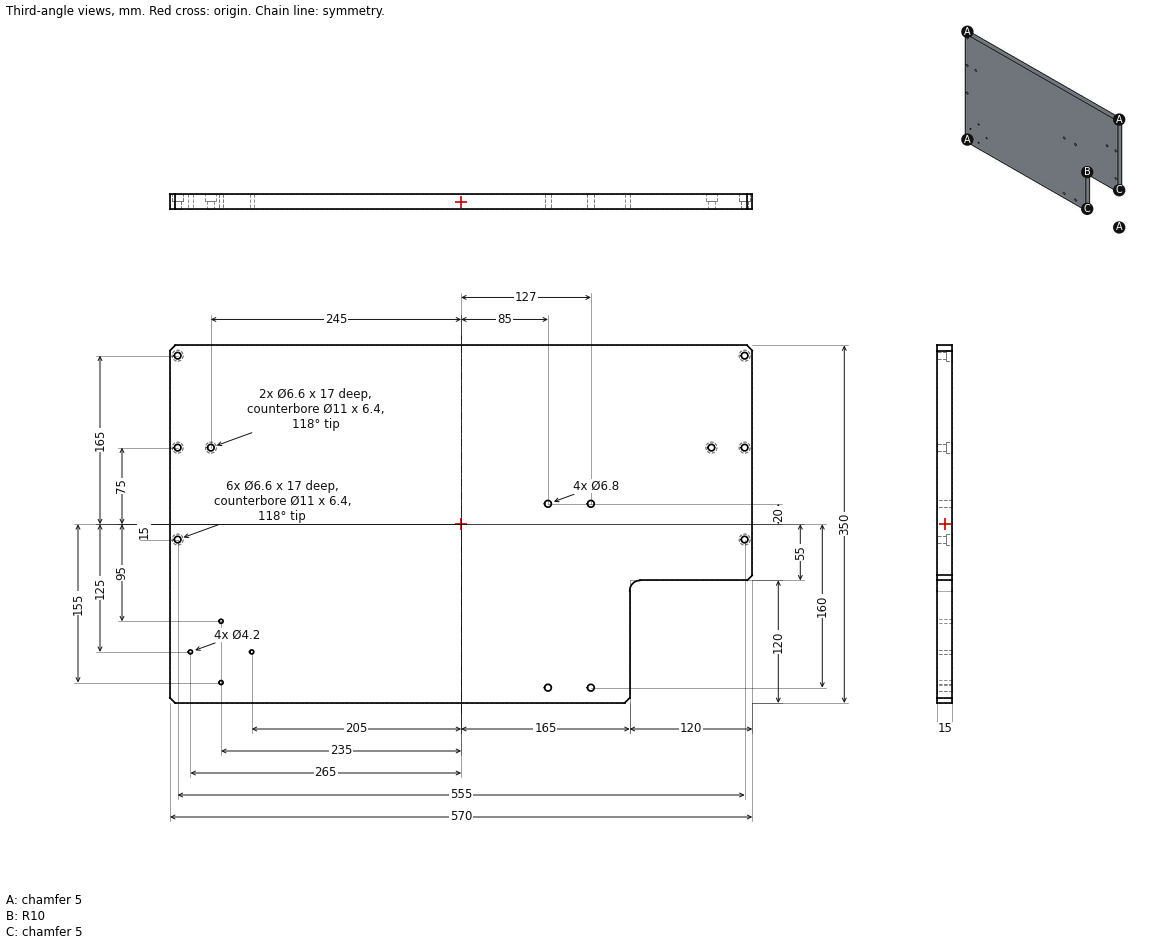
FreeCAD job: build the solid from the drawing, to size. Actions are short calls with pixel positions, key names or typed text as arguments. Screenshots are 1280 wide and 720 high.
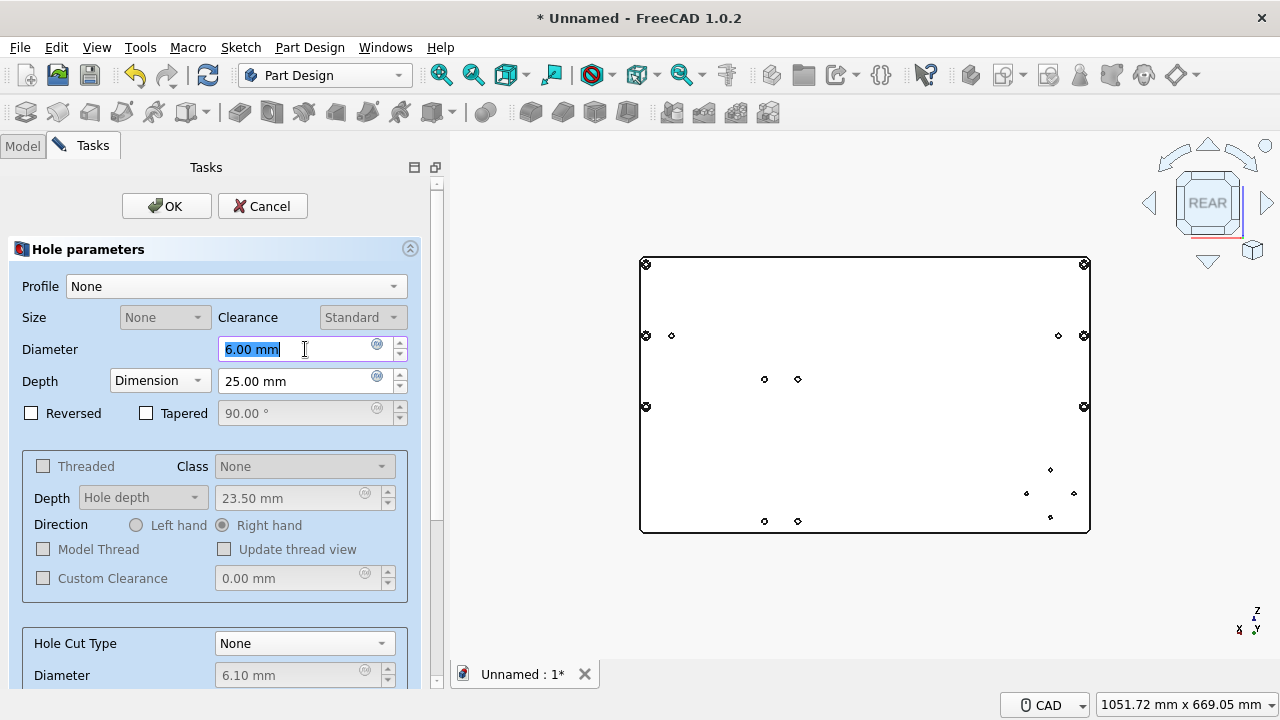
text(6.6)
key(Tab)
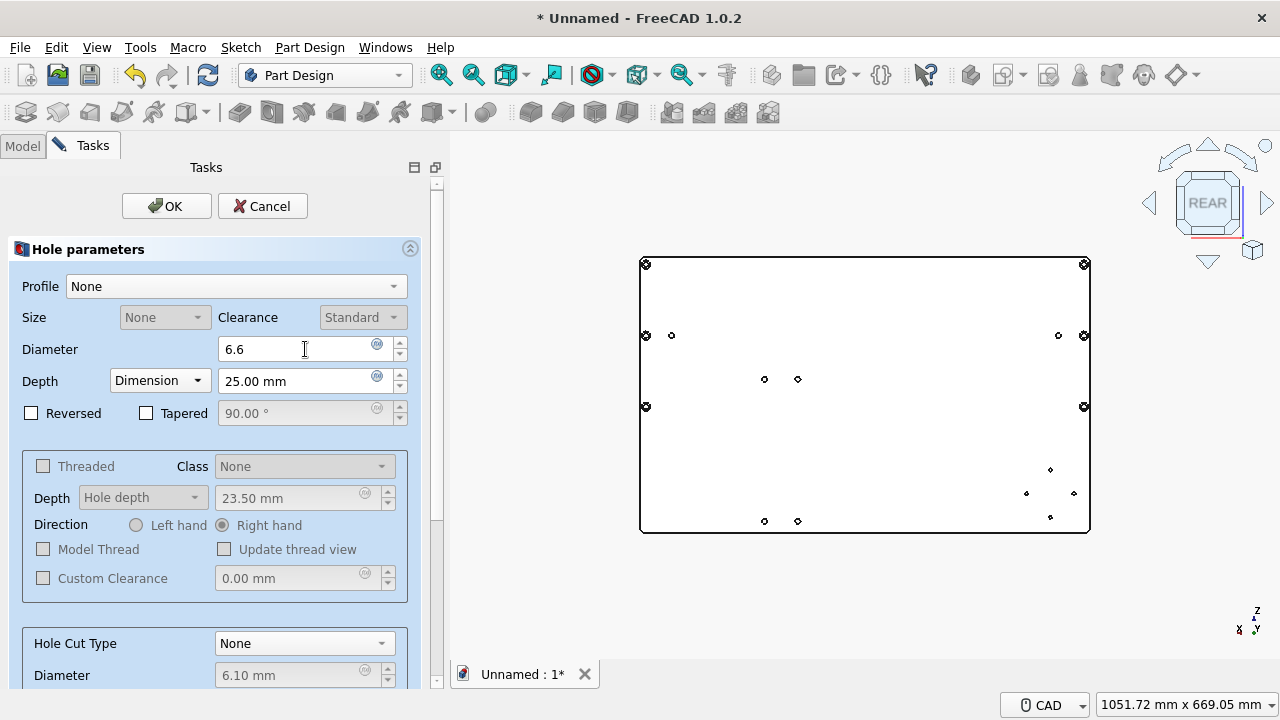
triple_click(305, 381)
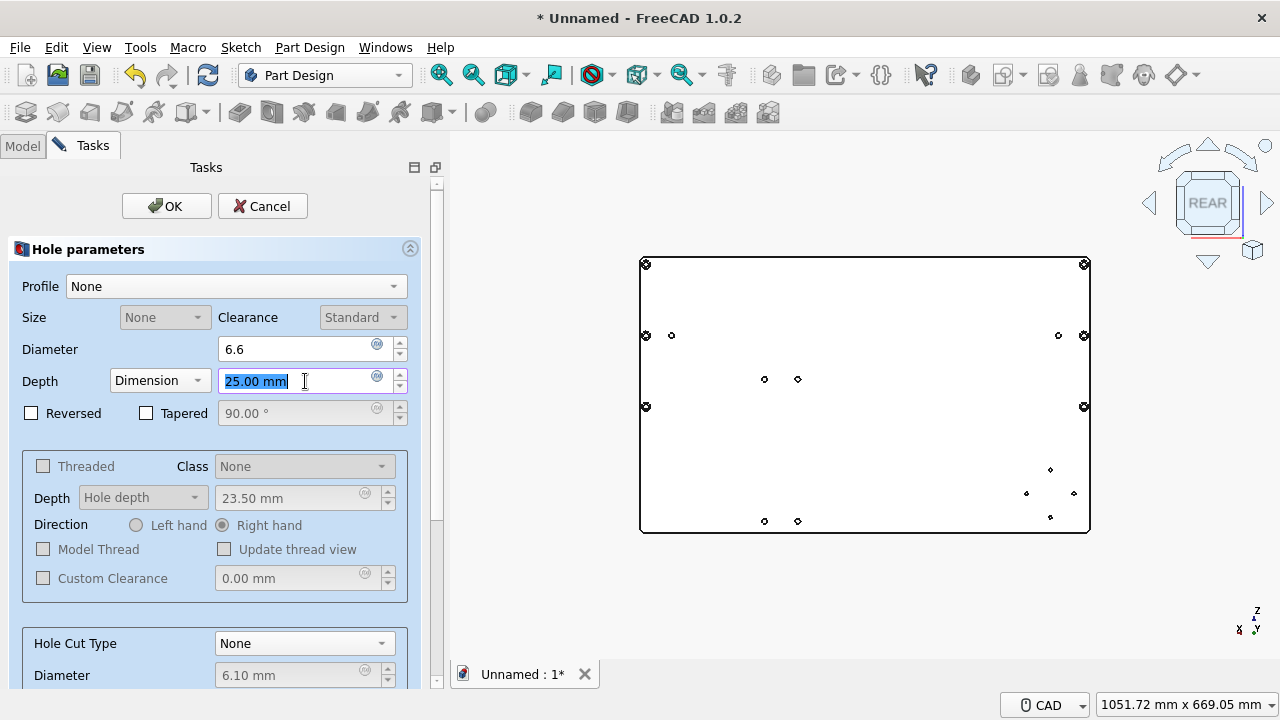
text(17)
key(Tab)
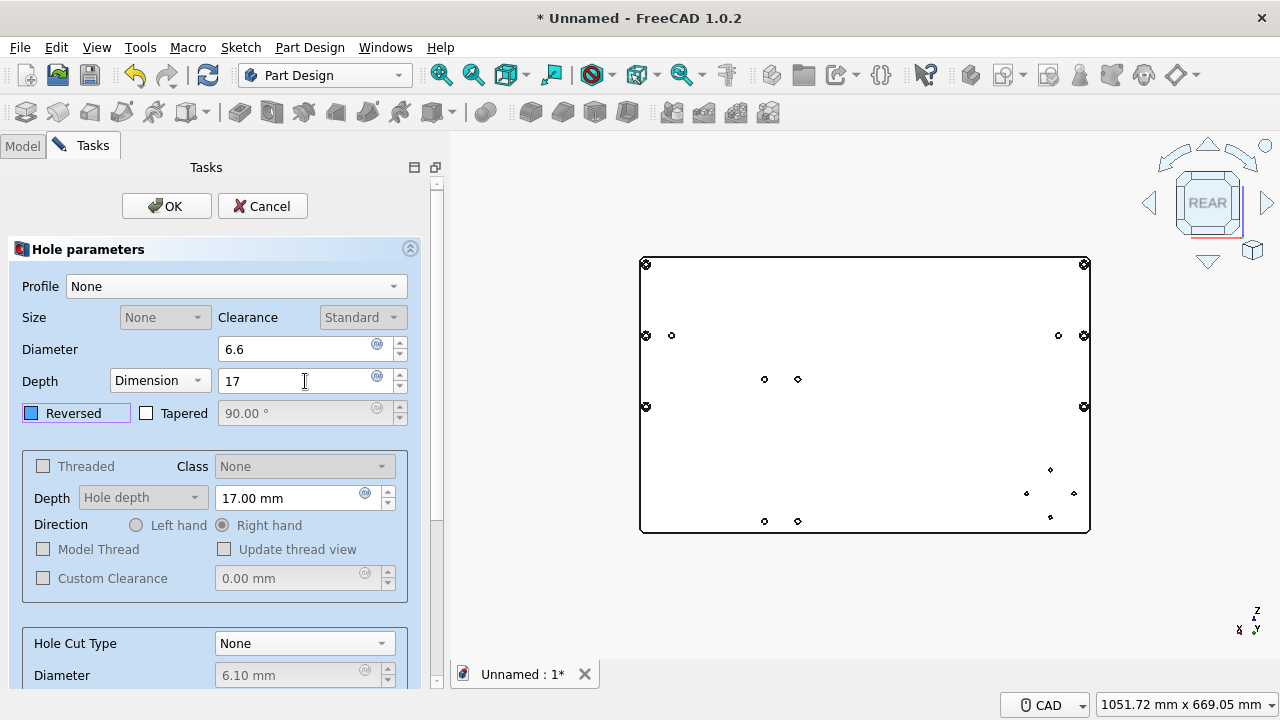
click(306, 644)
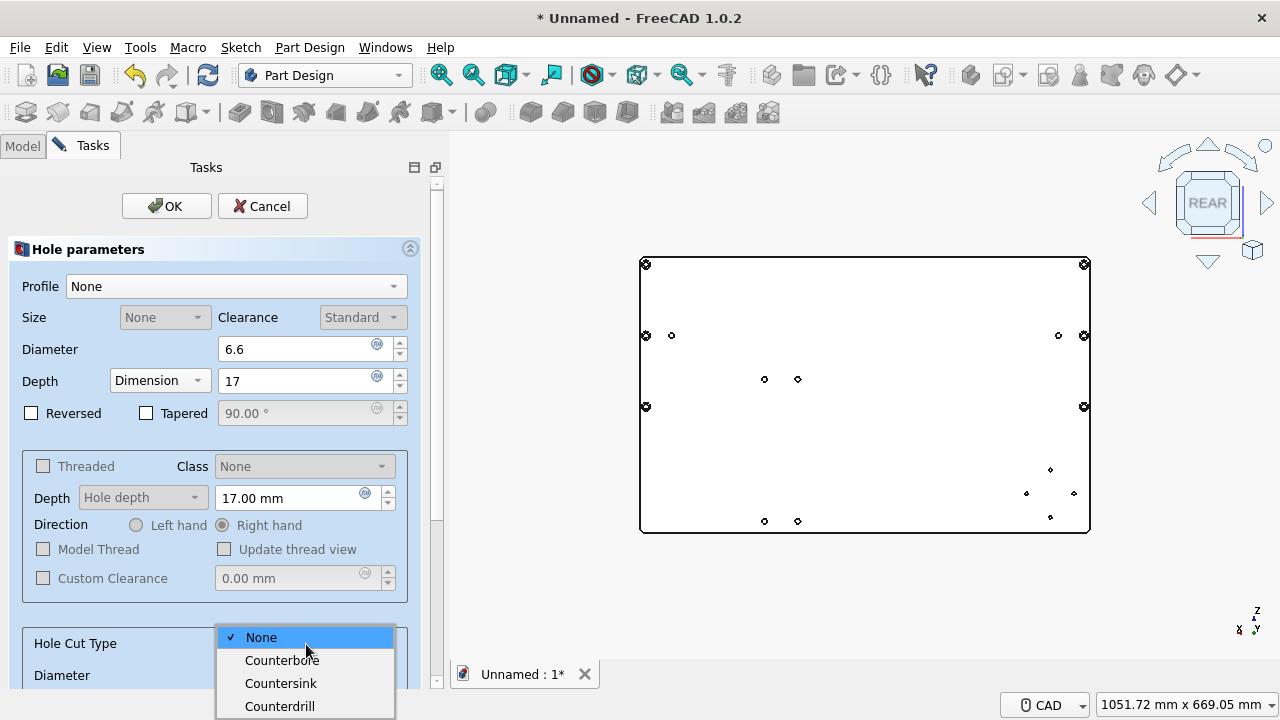
click(304, 660)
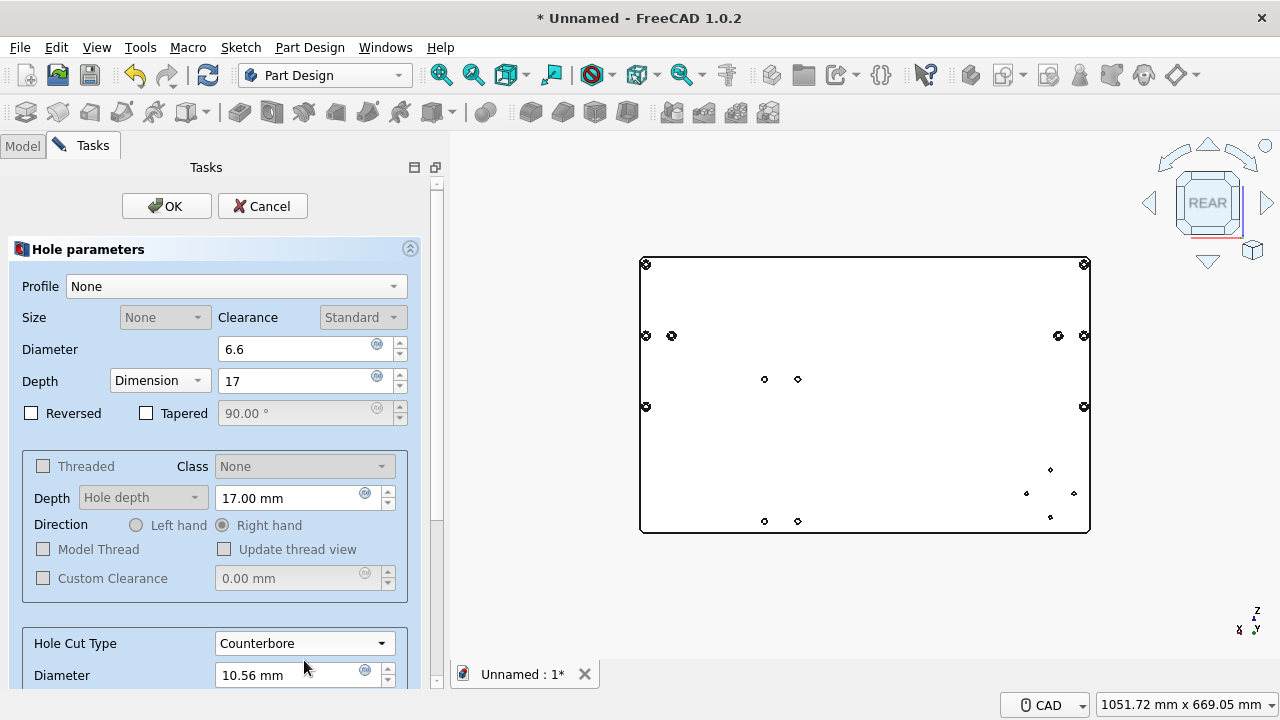
triple_click(298, 675)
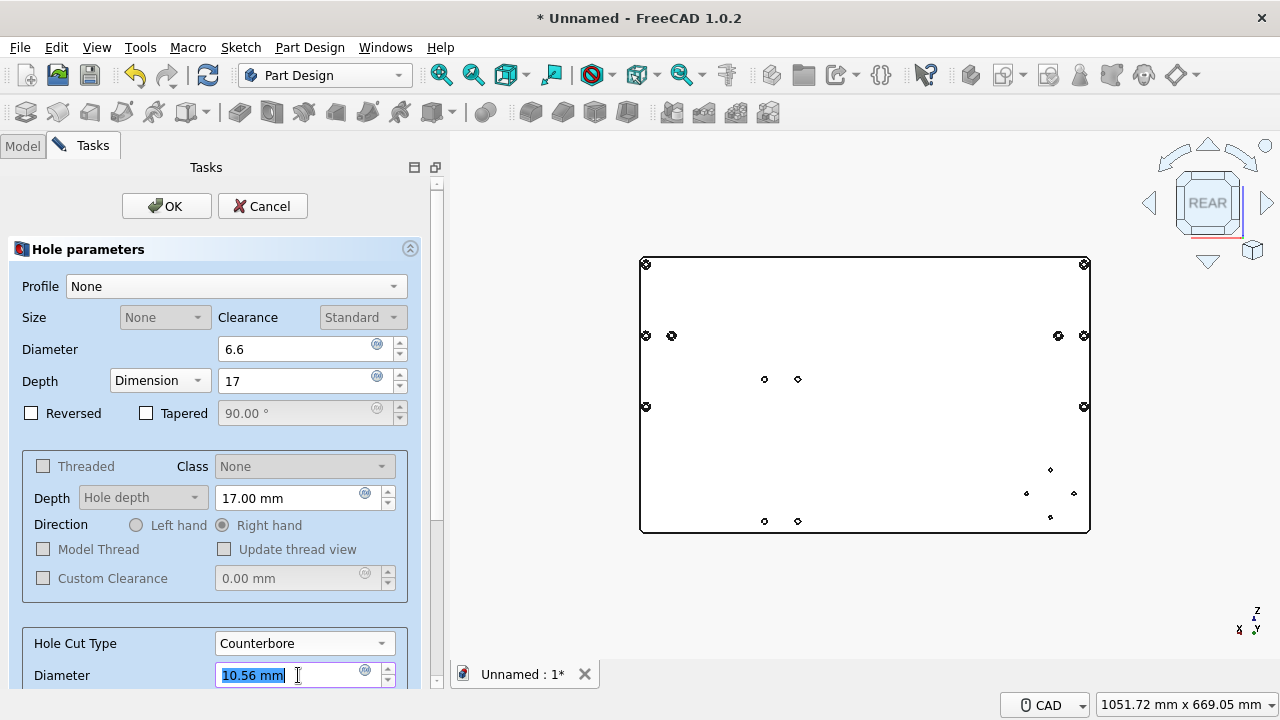
text(11)
key(Tab)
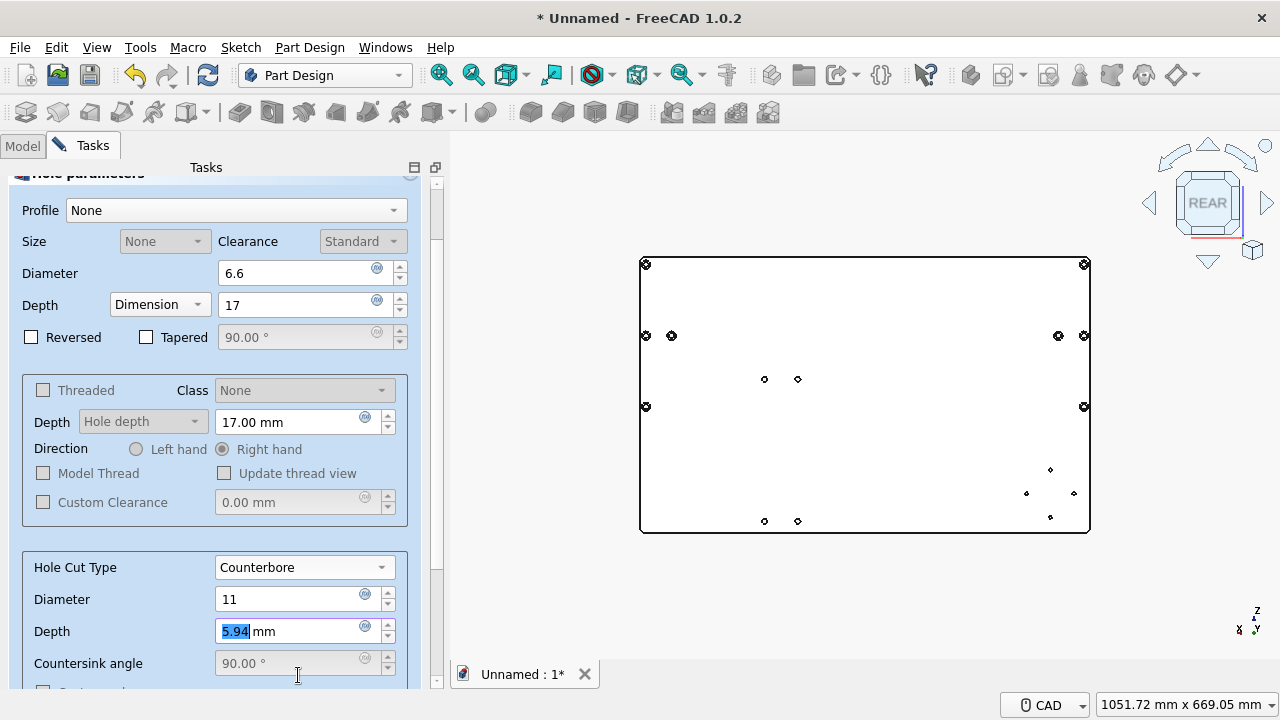
text(6.4)
key(Tab)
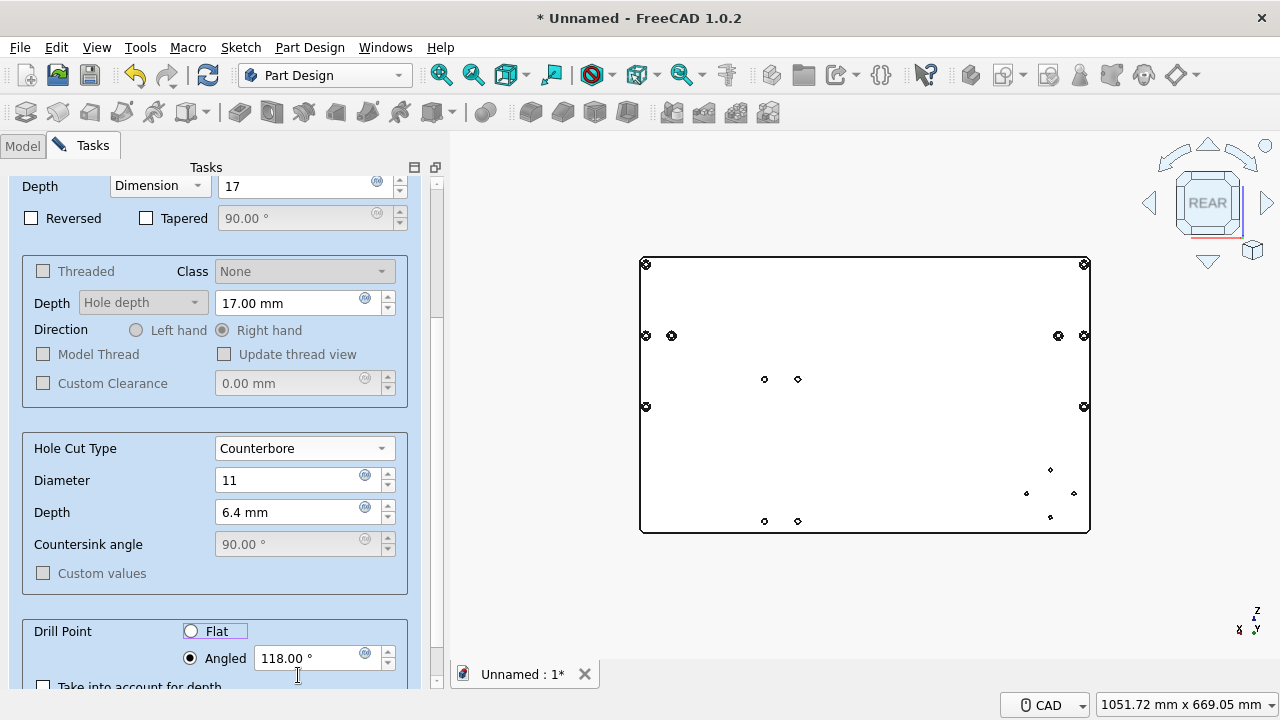
scroll(437, 432, up, 4)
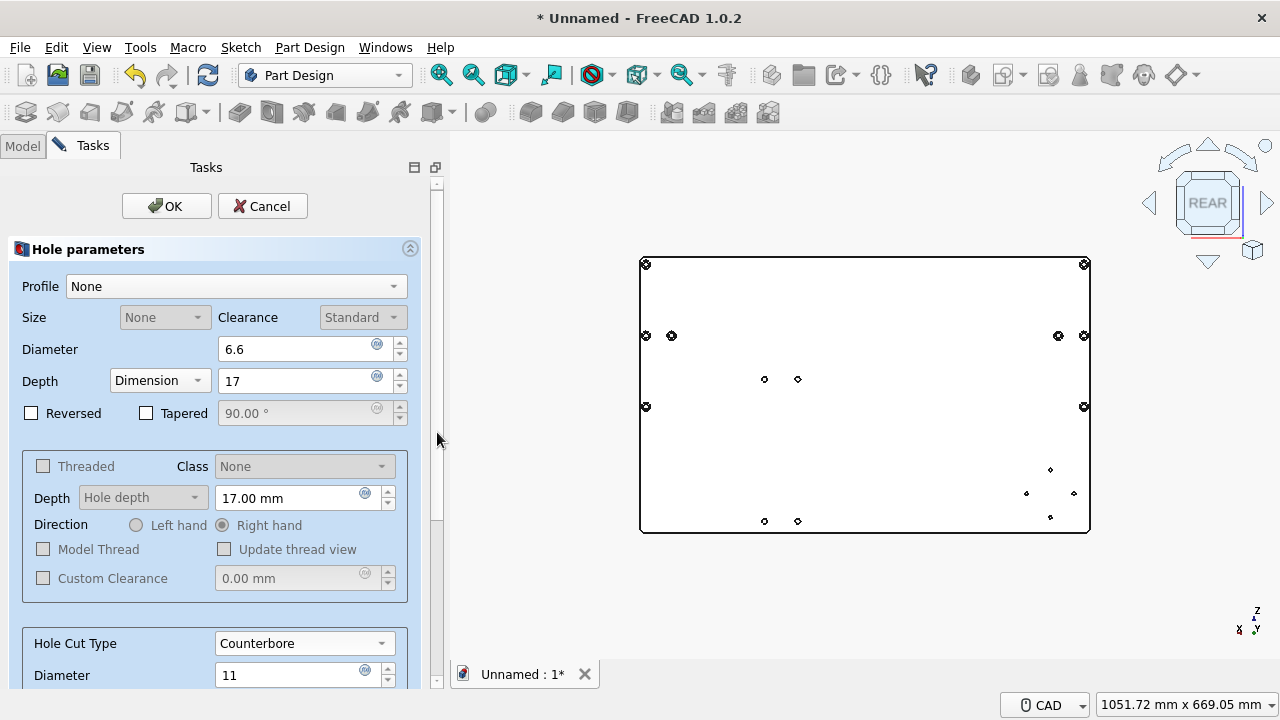
click(167, 206)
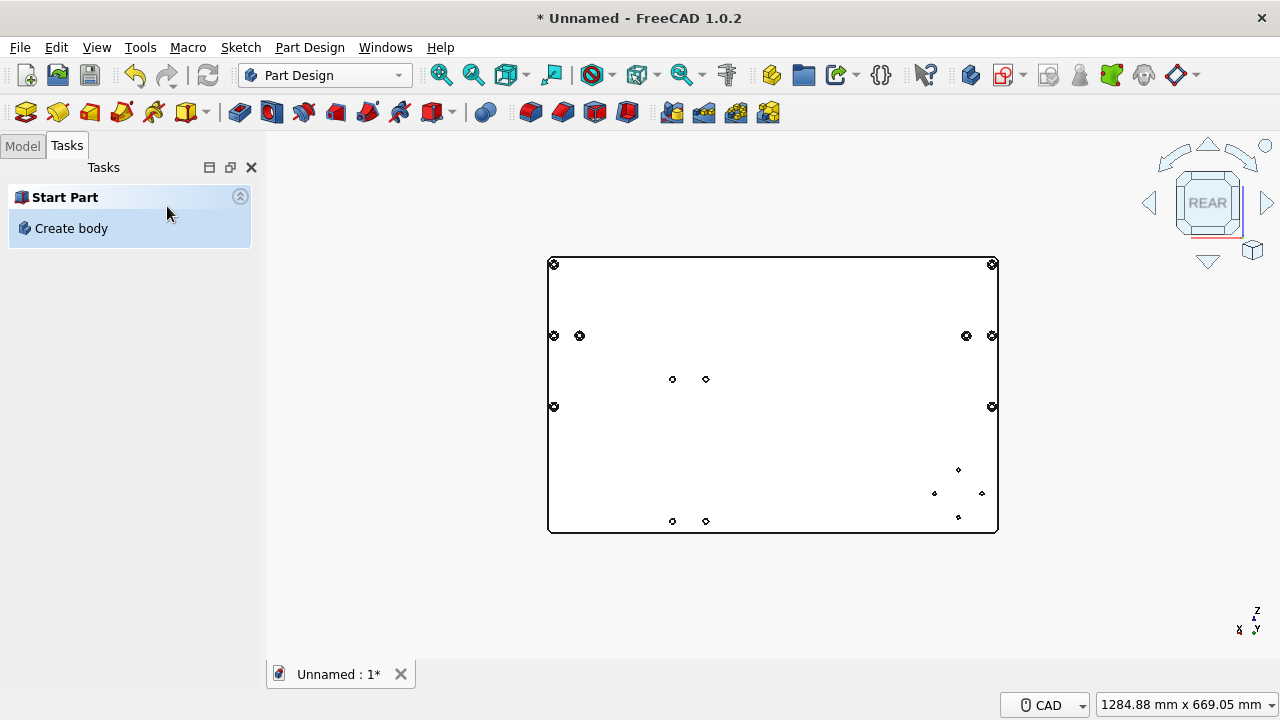
click(837, 394)